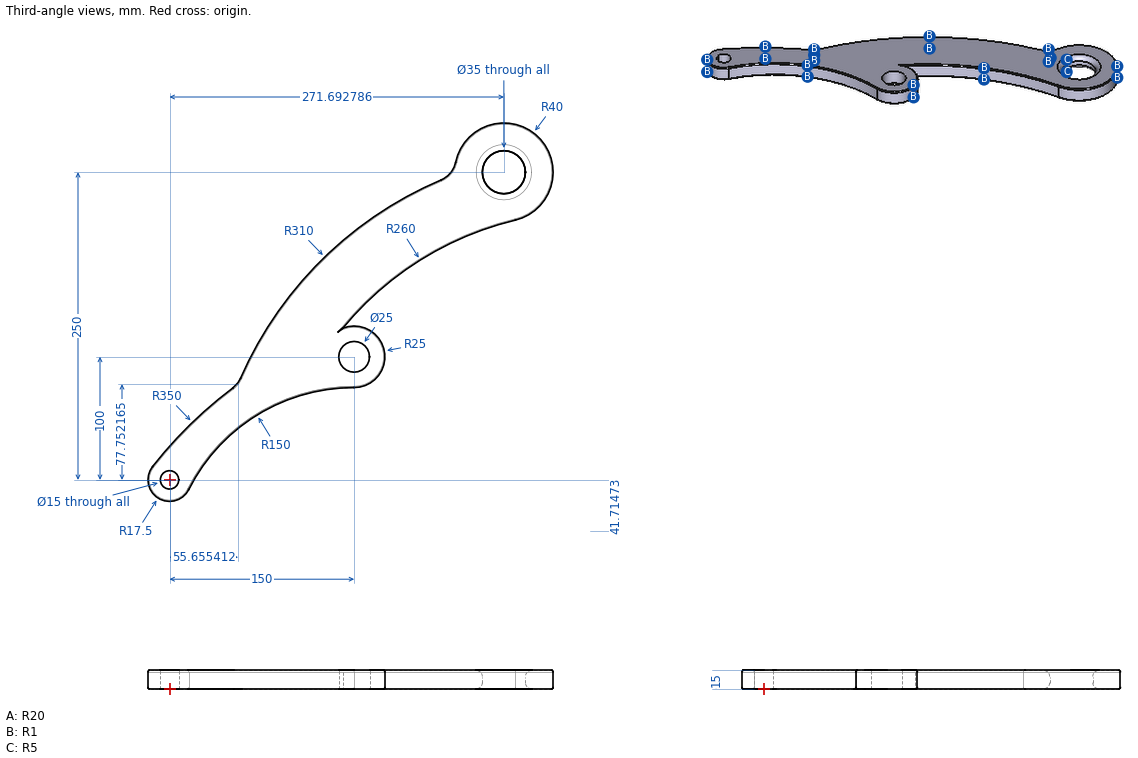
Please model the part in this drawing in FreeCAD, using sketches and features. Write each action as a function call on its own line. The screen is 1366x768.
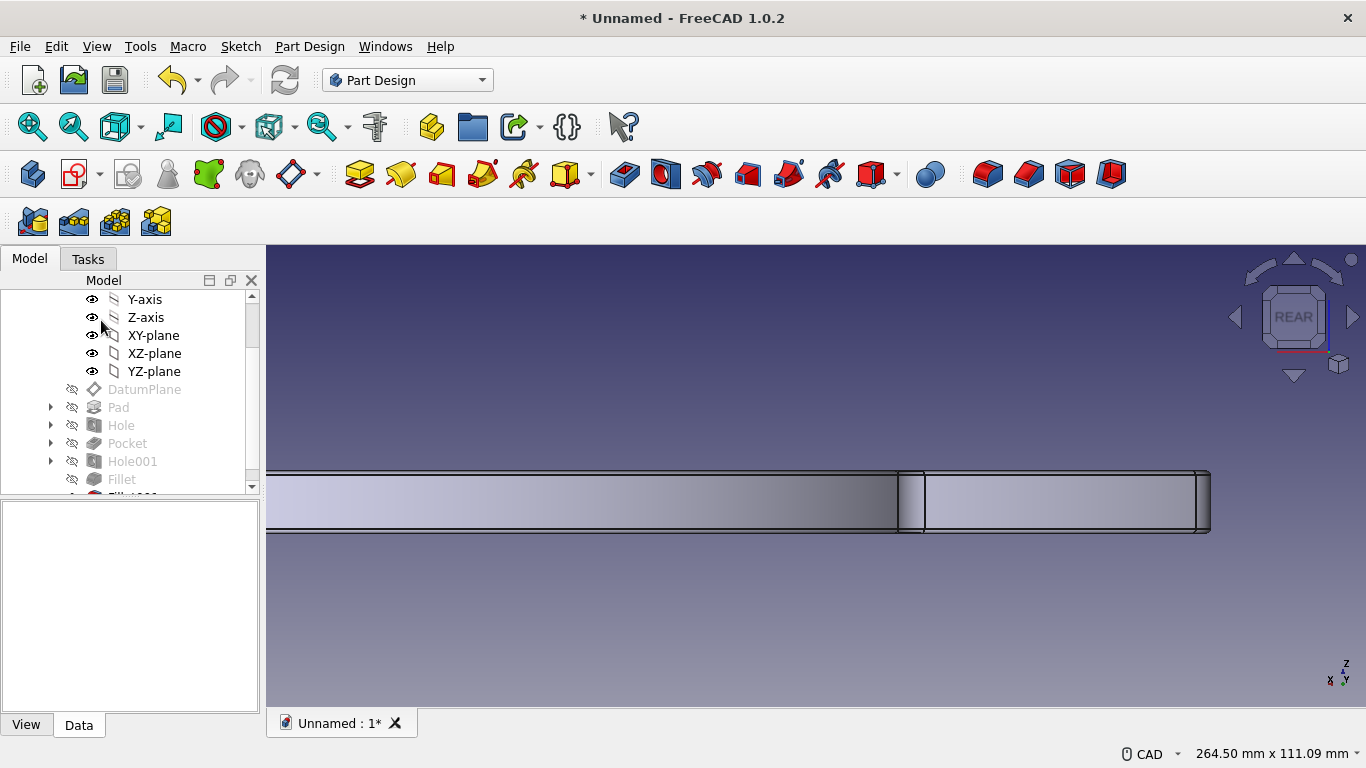
click(33, 128)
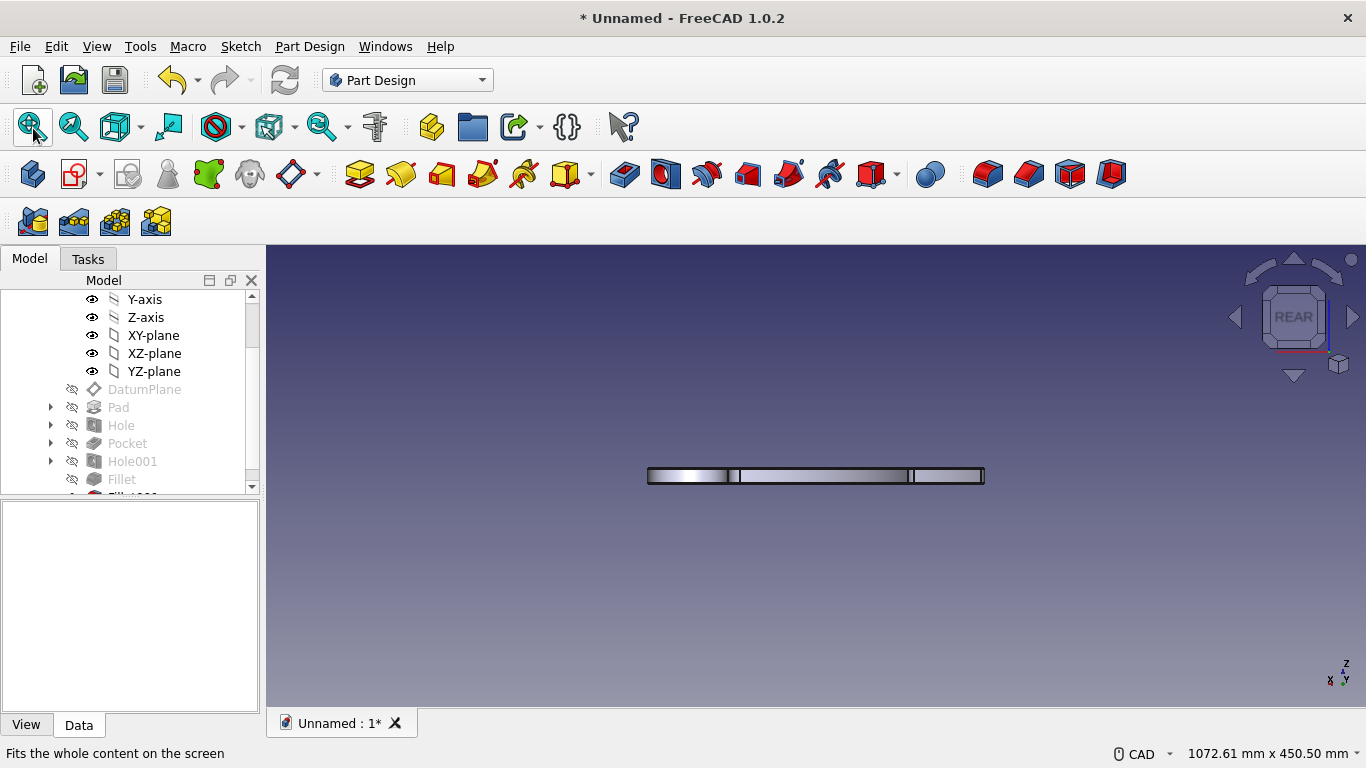
key(0)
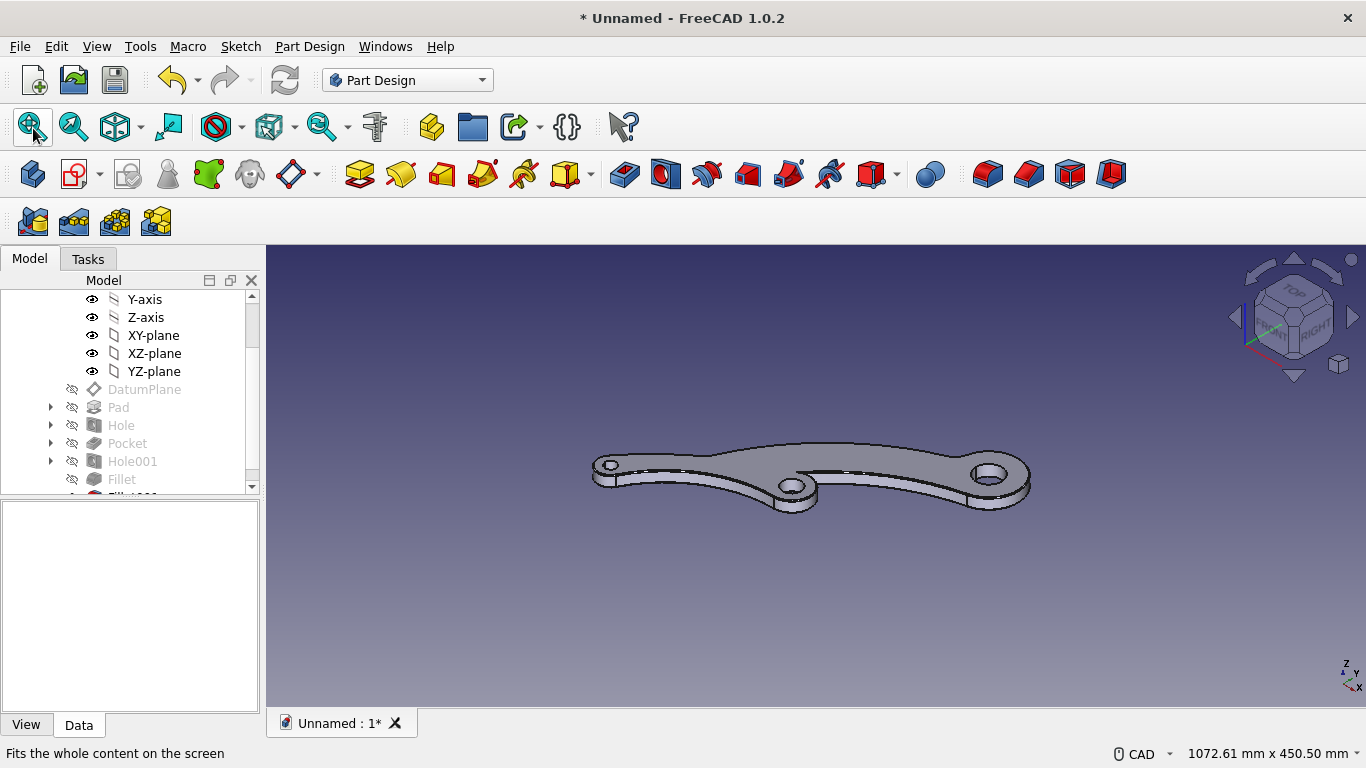
click(1007, 475)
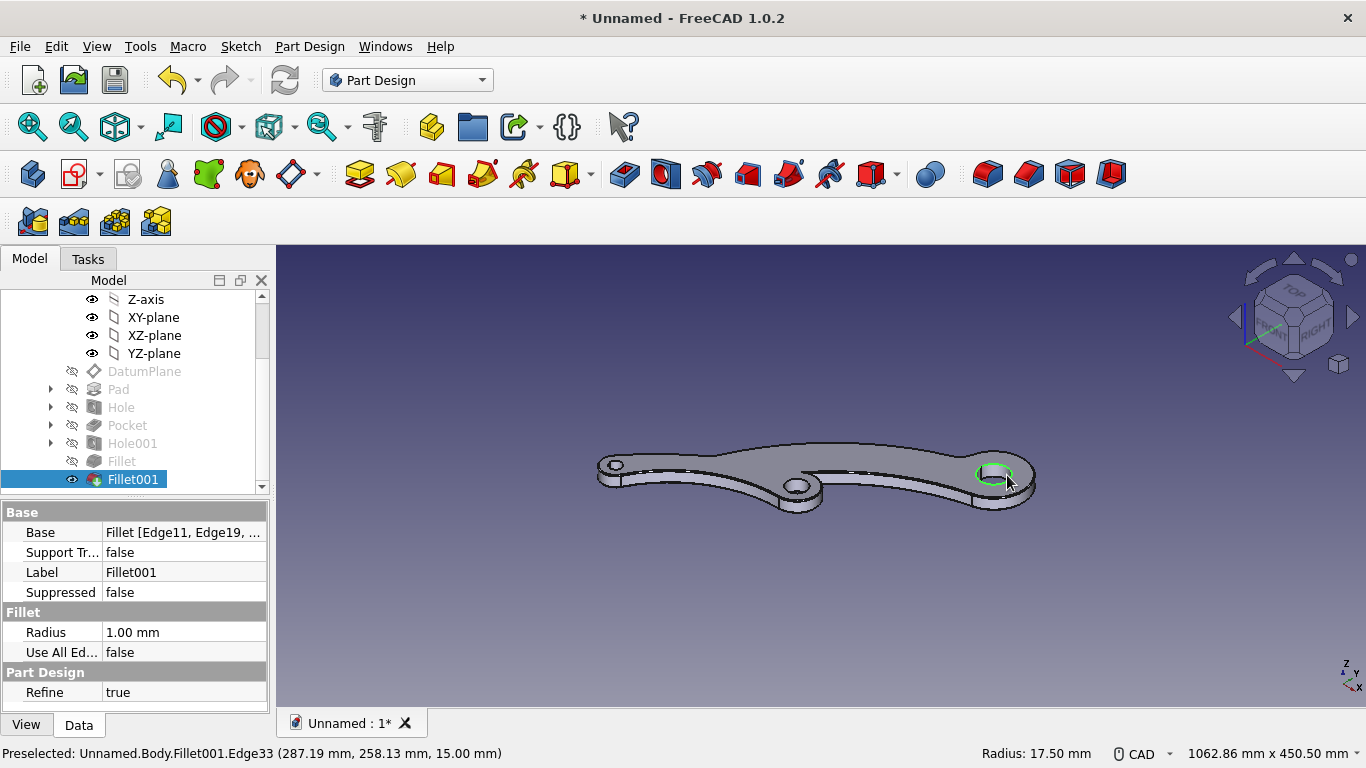
key(2)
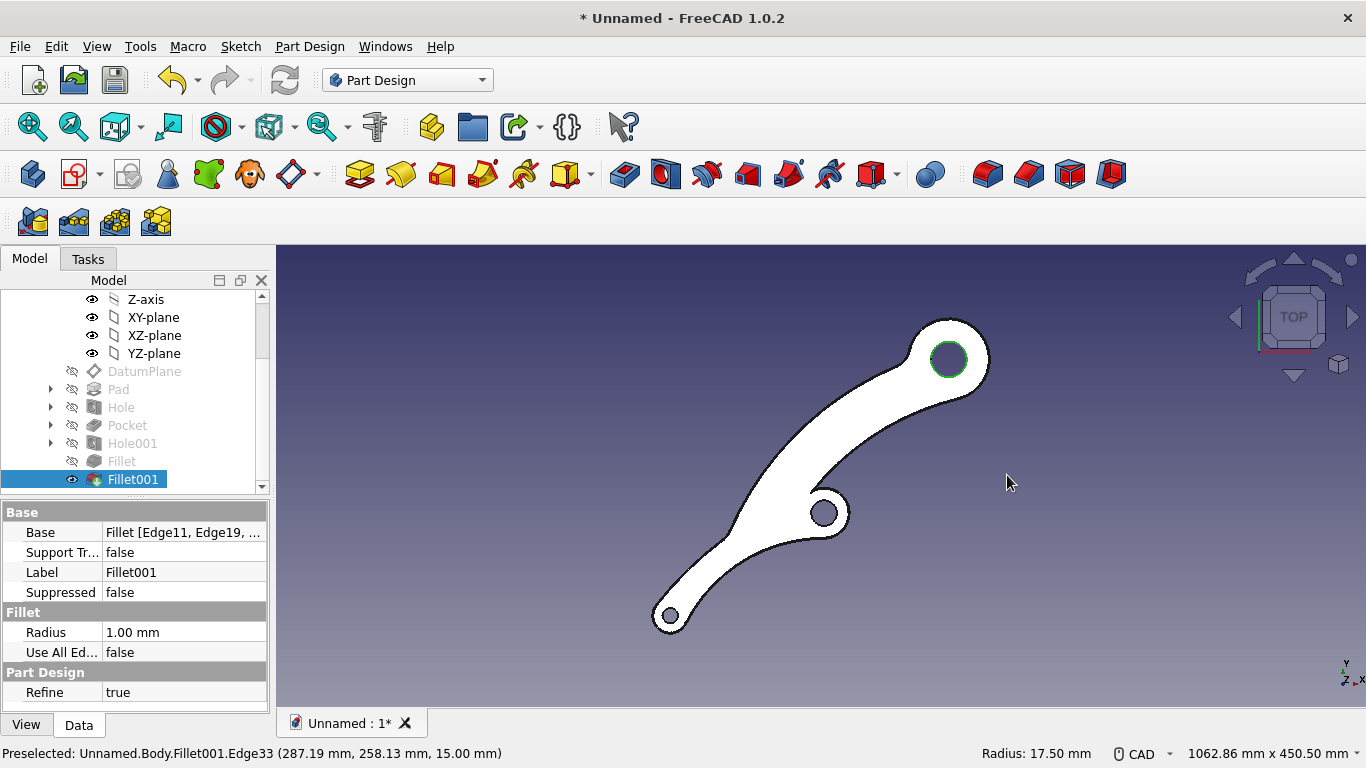
key(1)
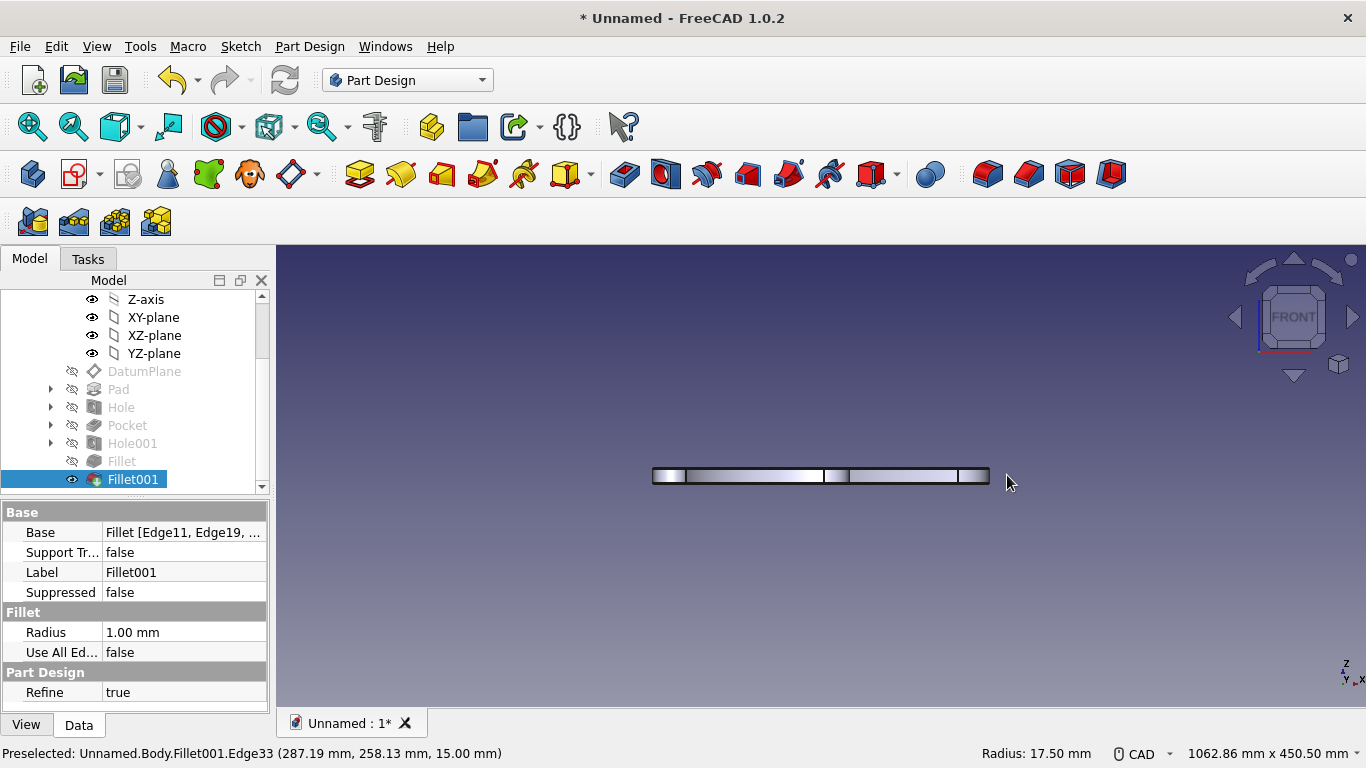
click(33, 128)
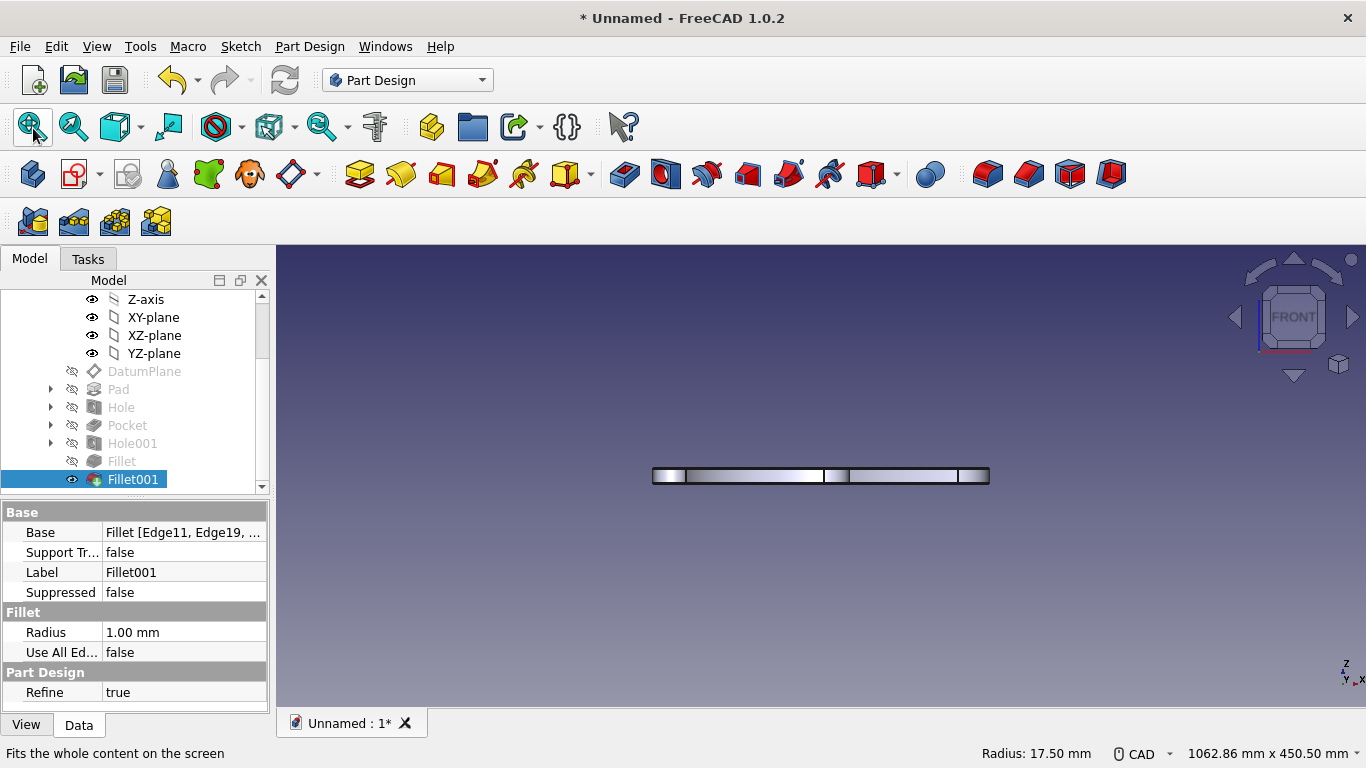
key(3)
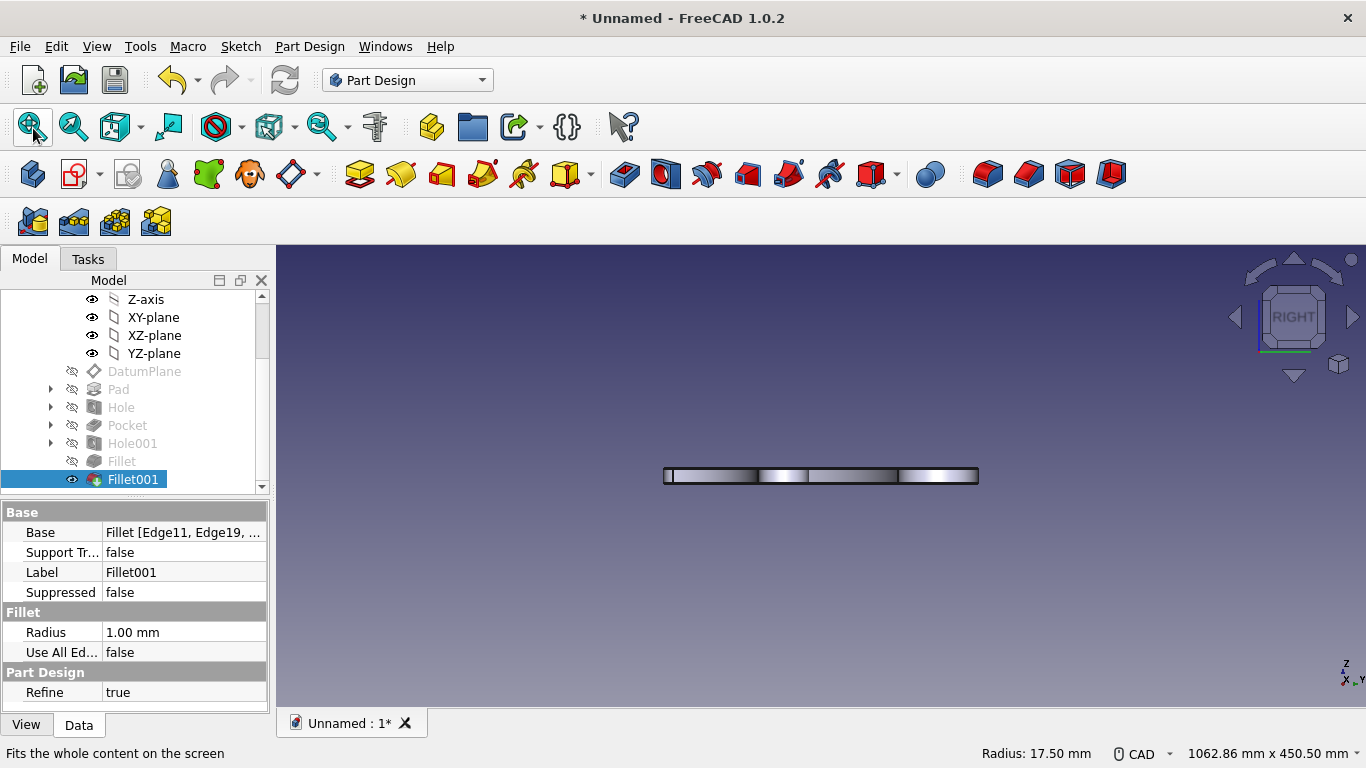
click(33, 128)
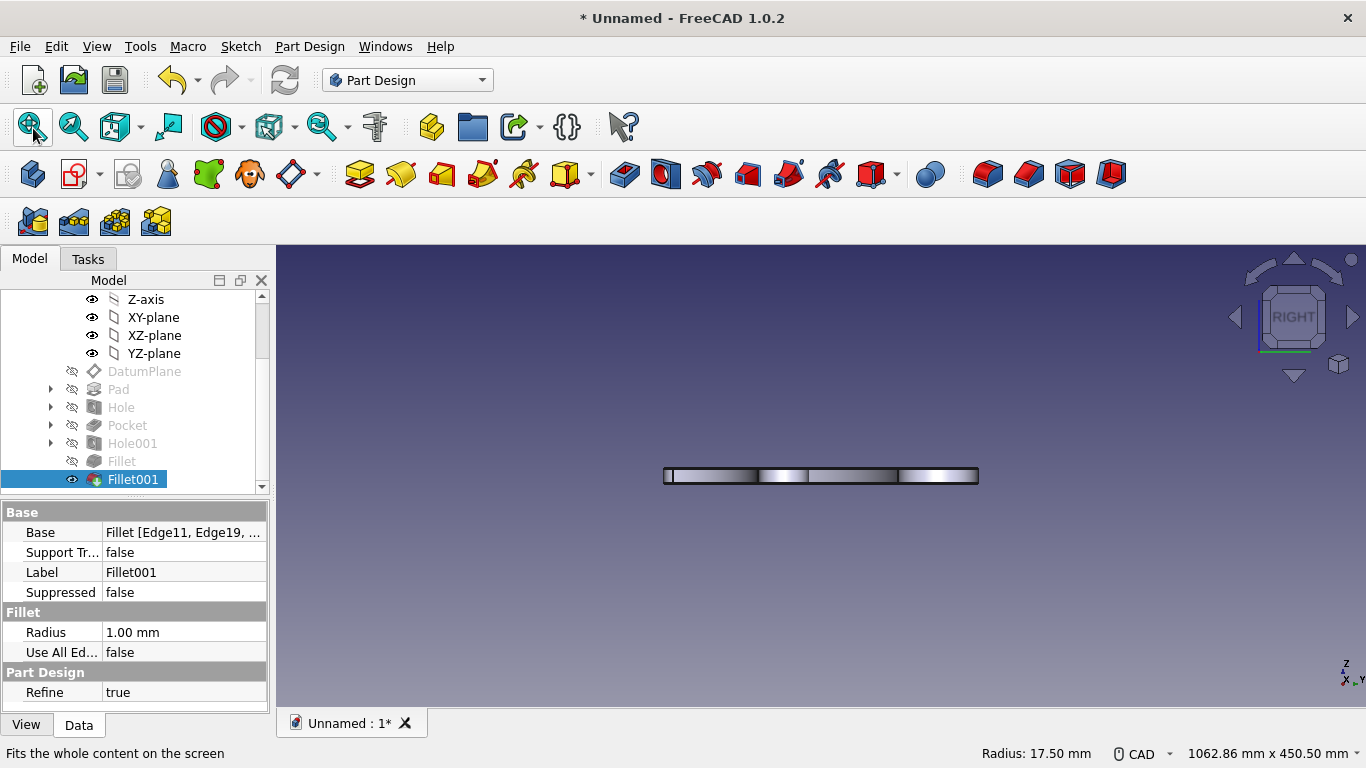
key(5)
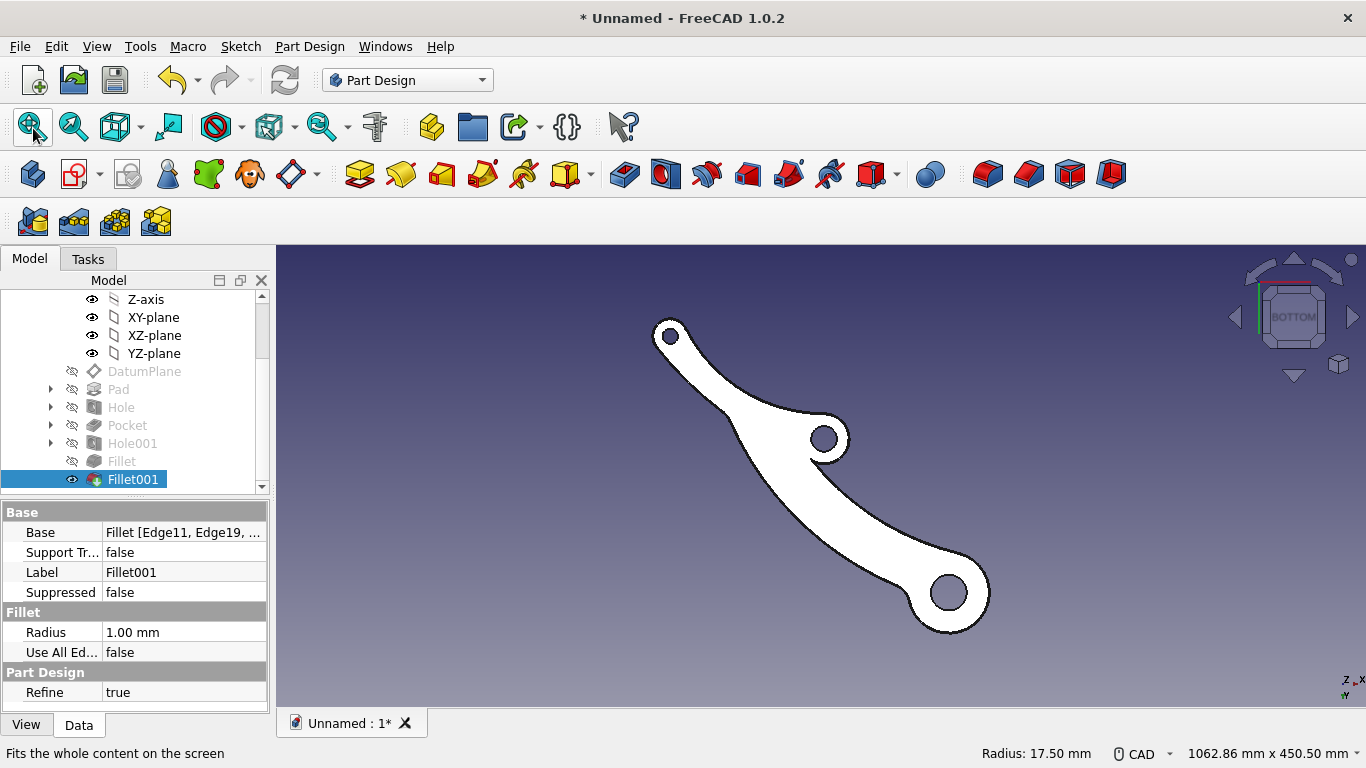
click(967, 592, ctrl)